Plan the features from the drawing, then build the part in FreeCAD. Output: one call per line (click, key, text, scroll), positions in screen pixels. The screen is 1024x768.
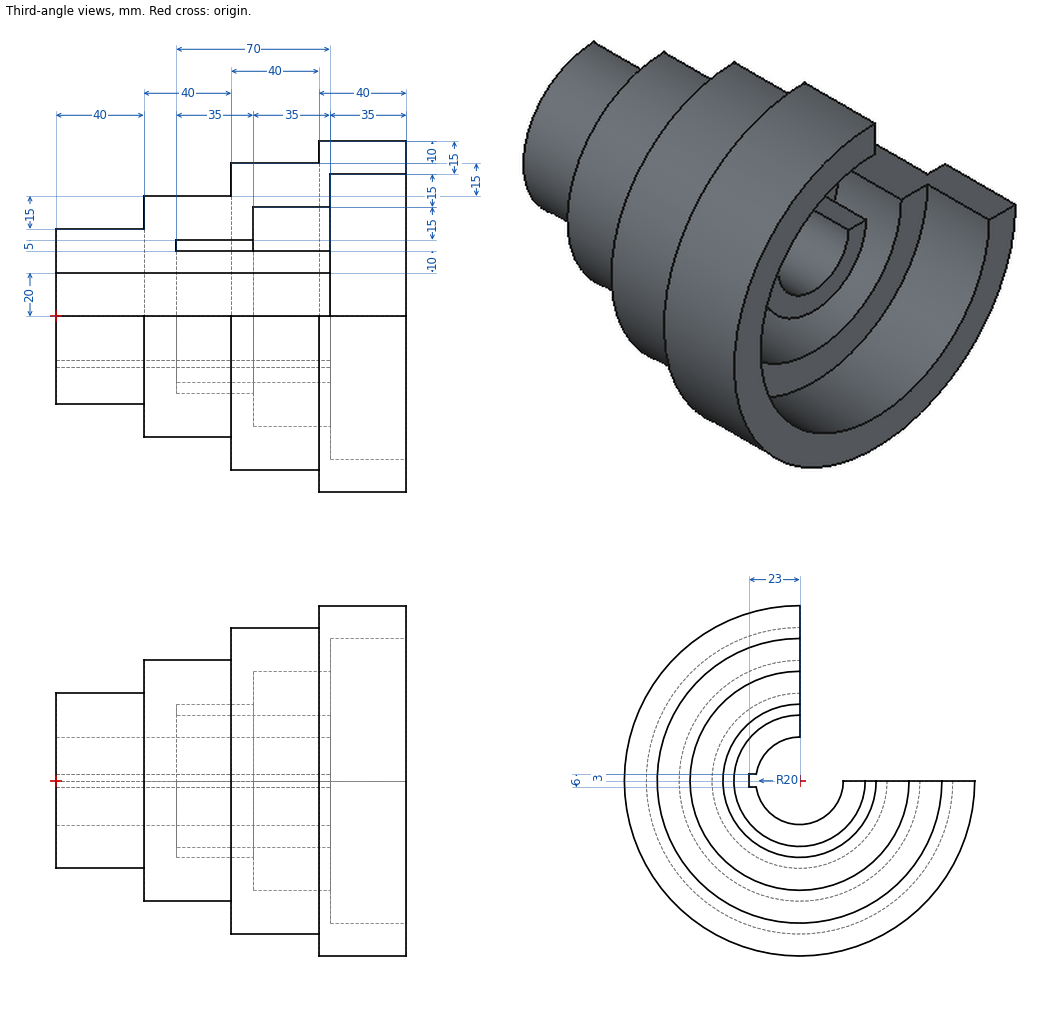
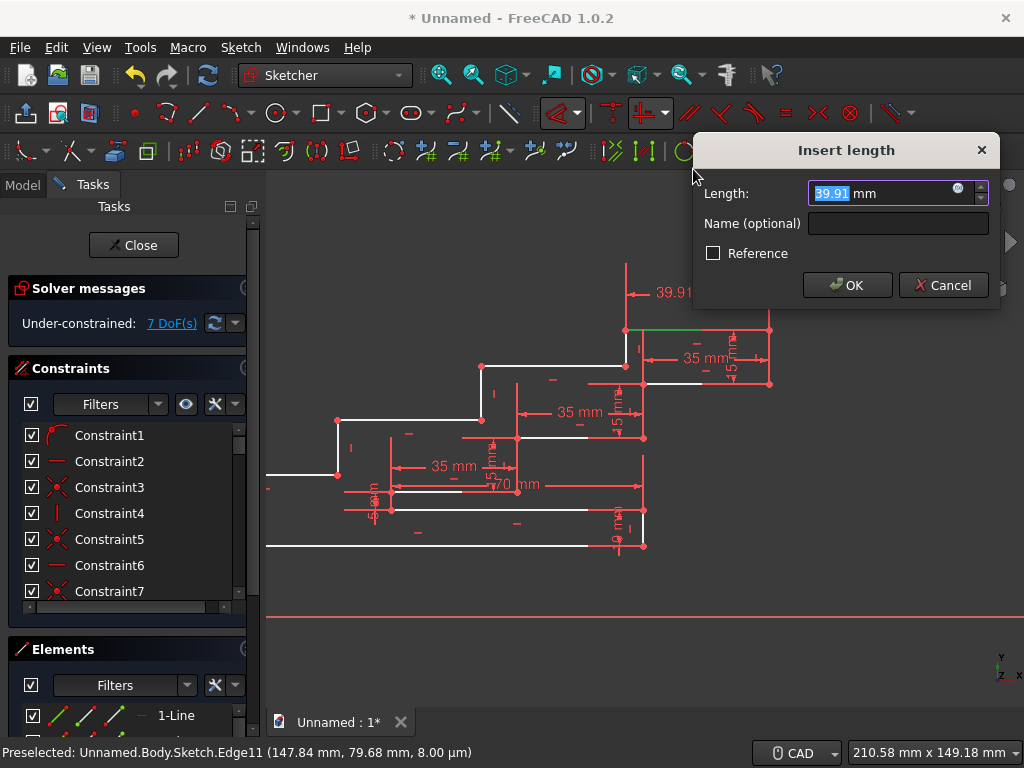
text(40)
key(Return)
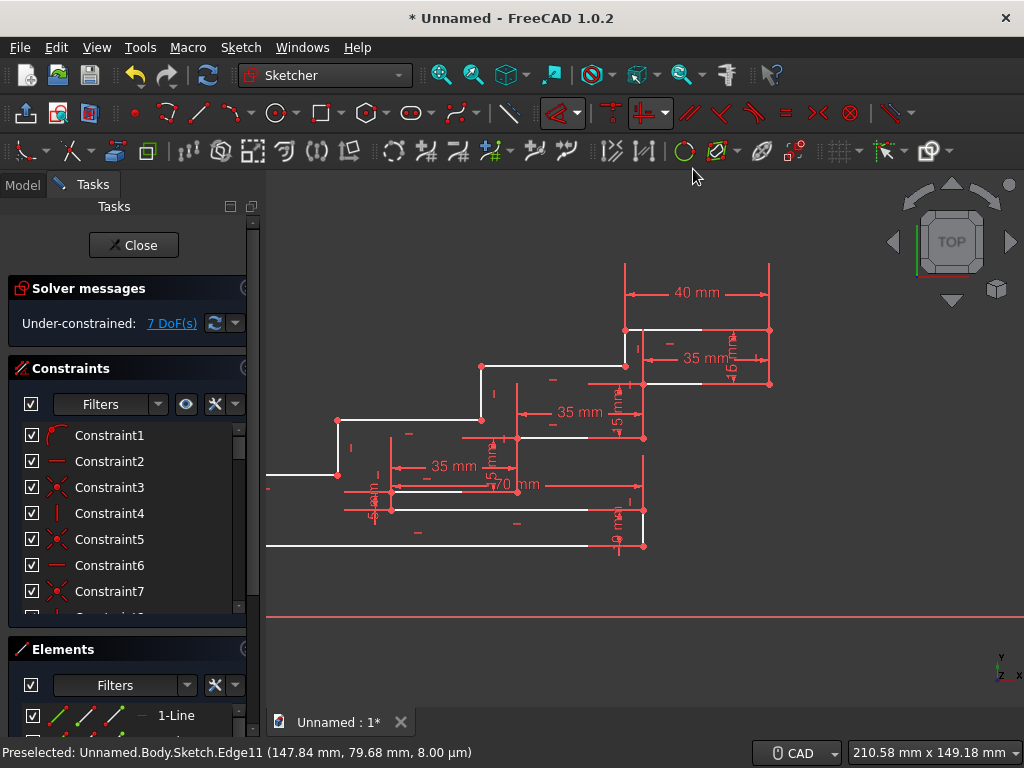
scroll(625, 341, up, 2)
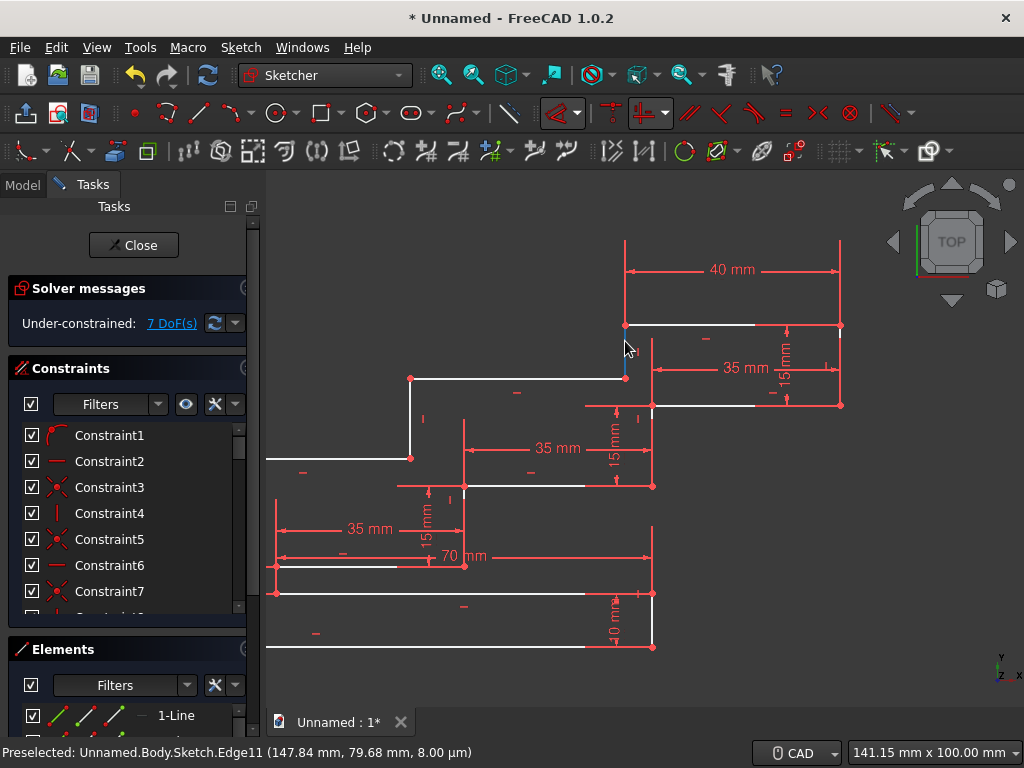
click(625, 341)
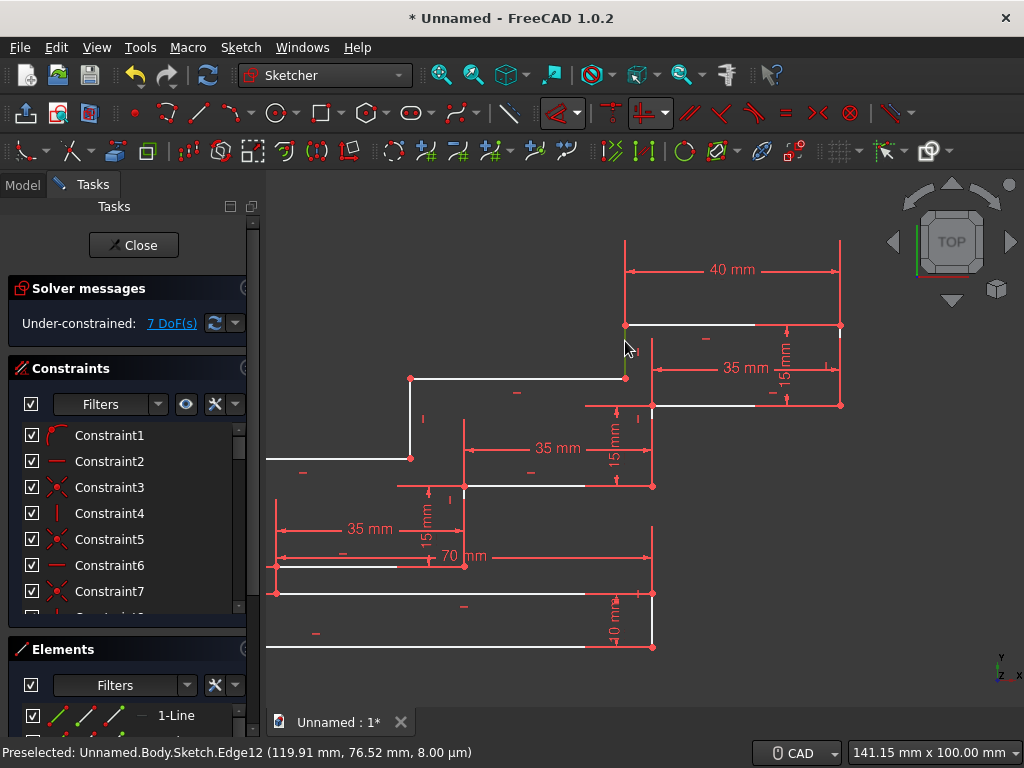
click(580, 114)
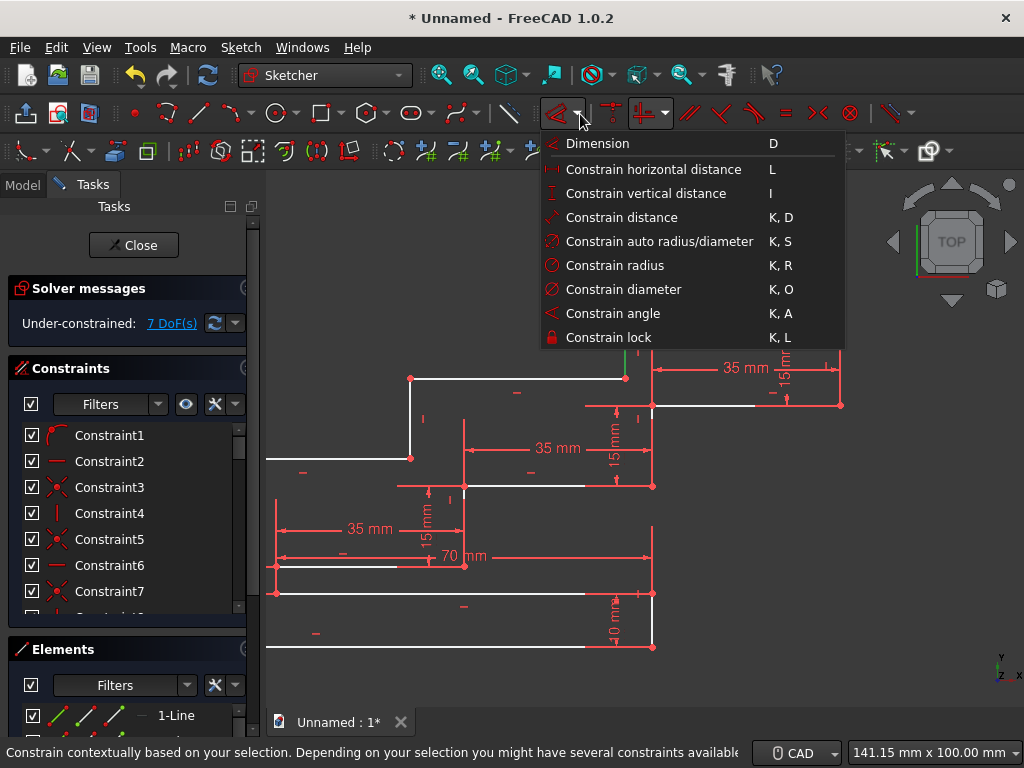
click(693, 193)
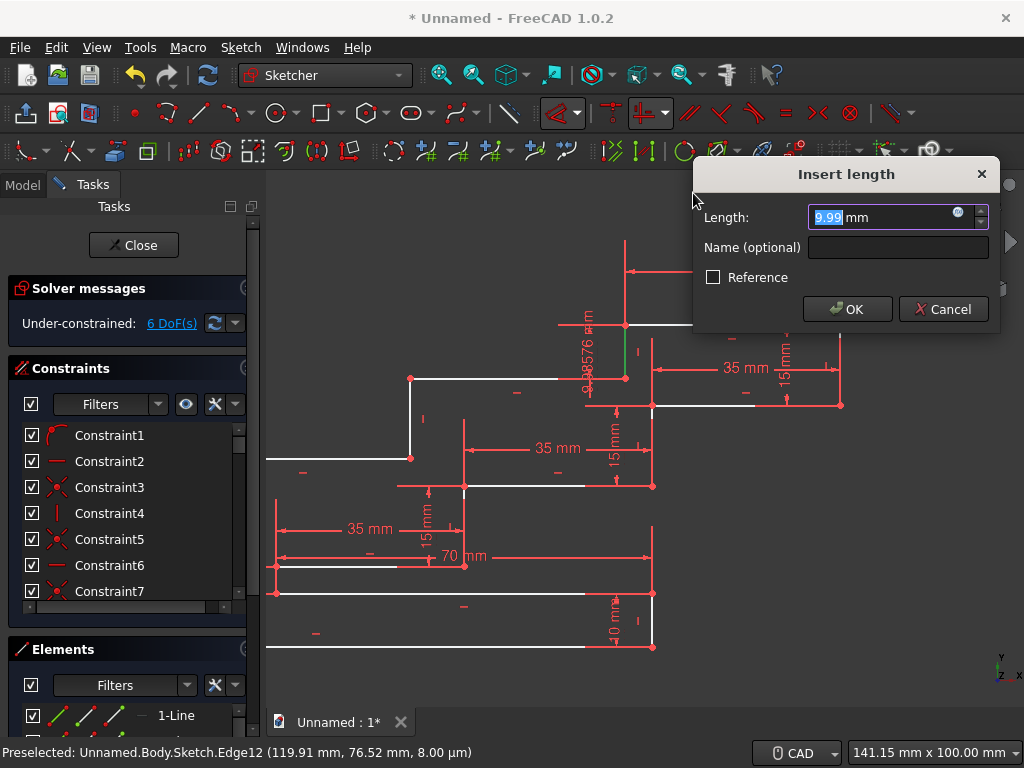
text(10)
key(Return)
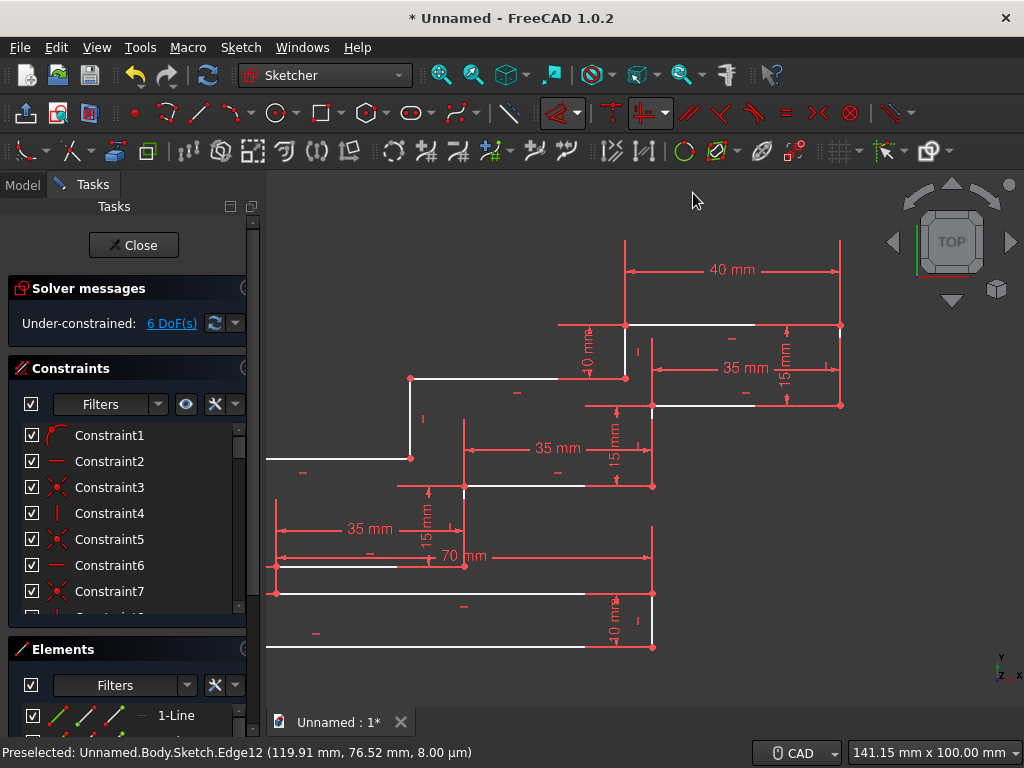
click(561, 379)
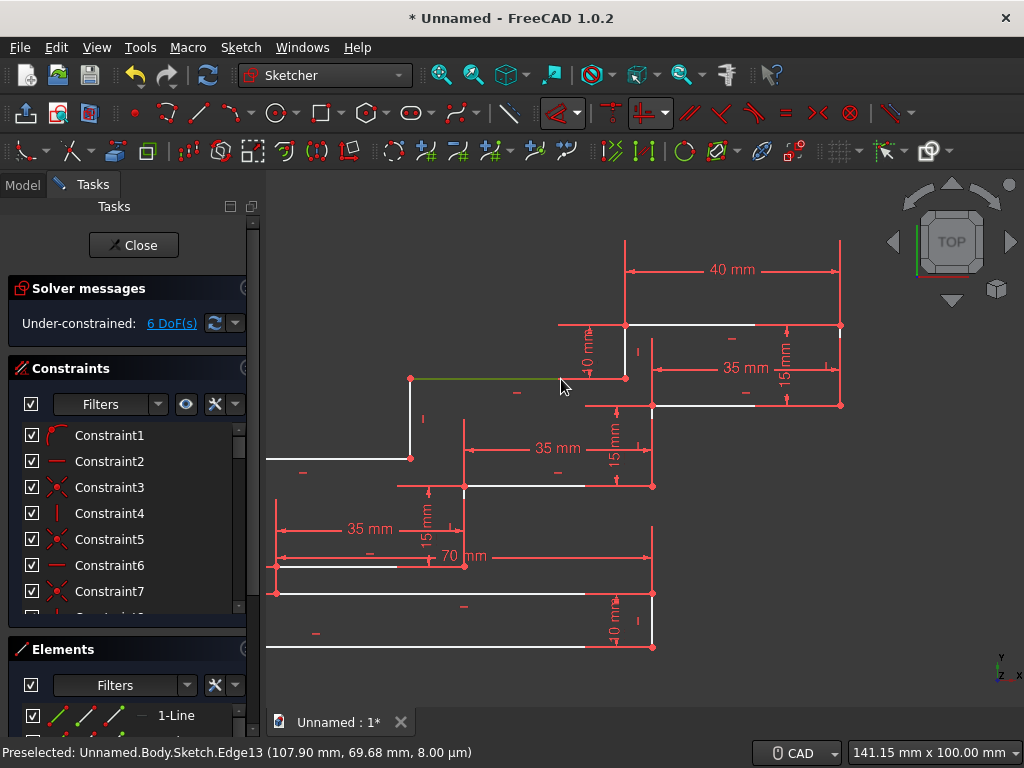
key(l)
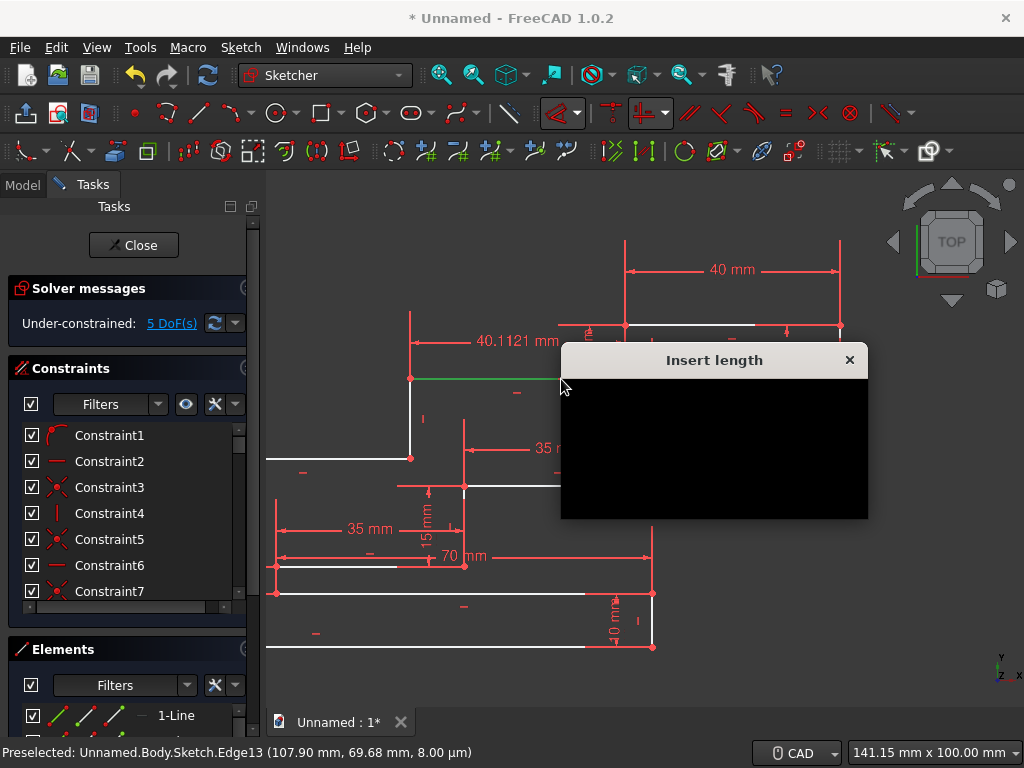
text(40)
key(Return)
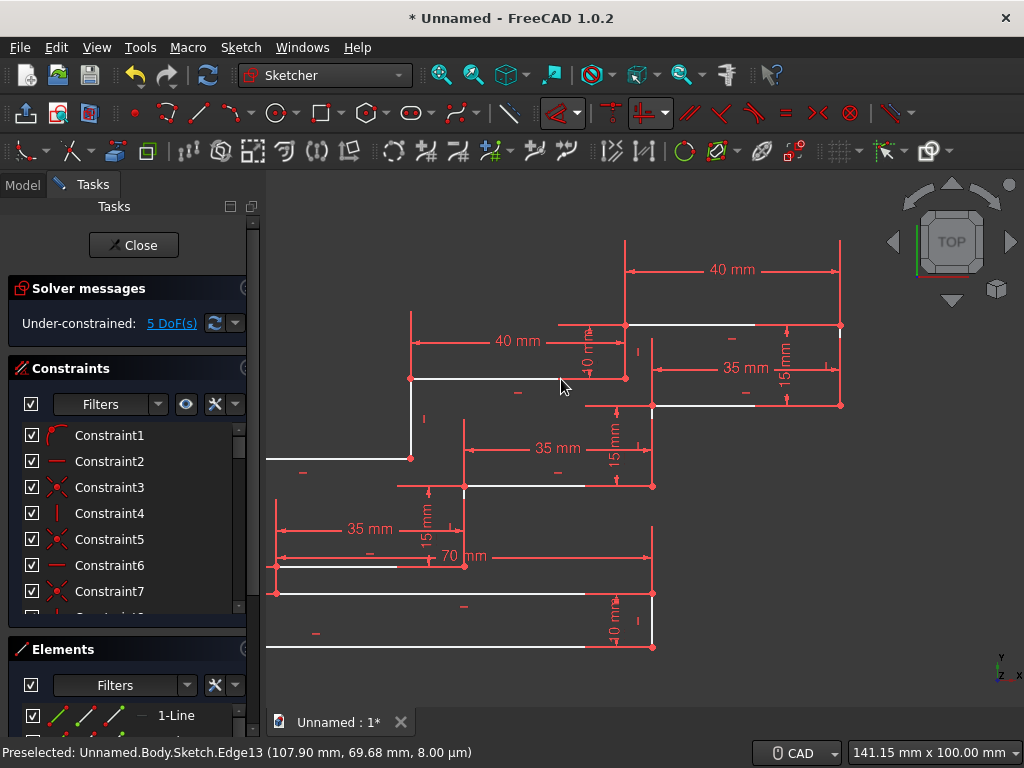
click(411, 403)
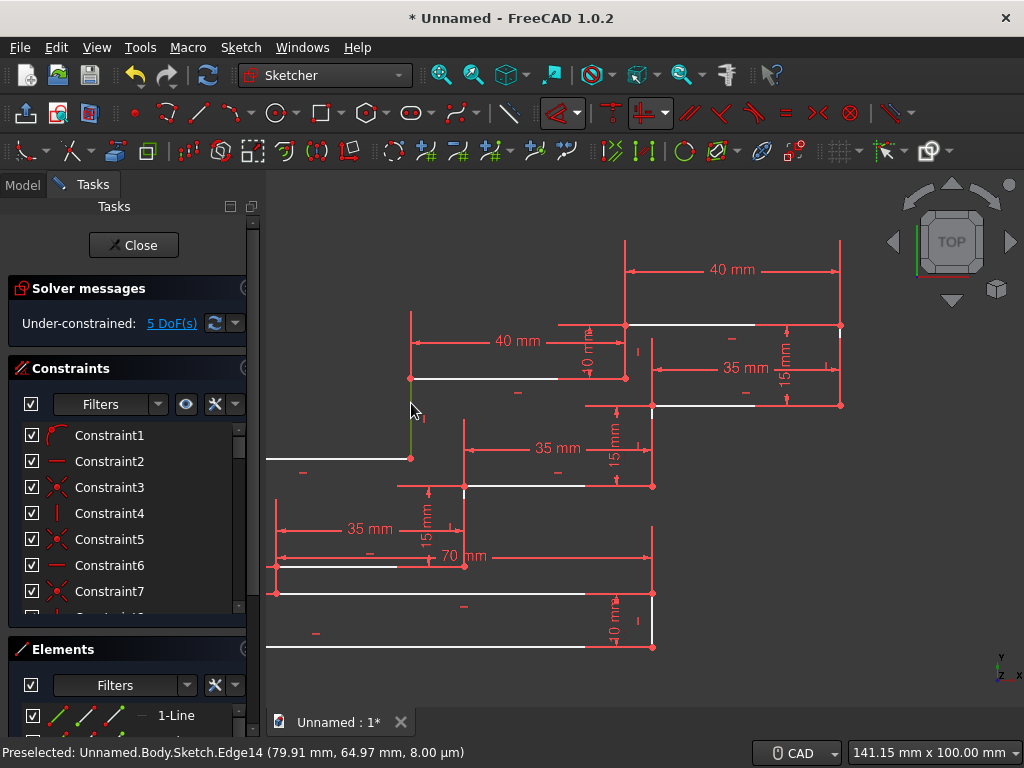
click(580, 114)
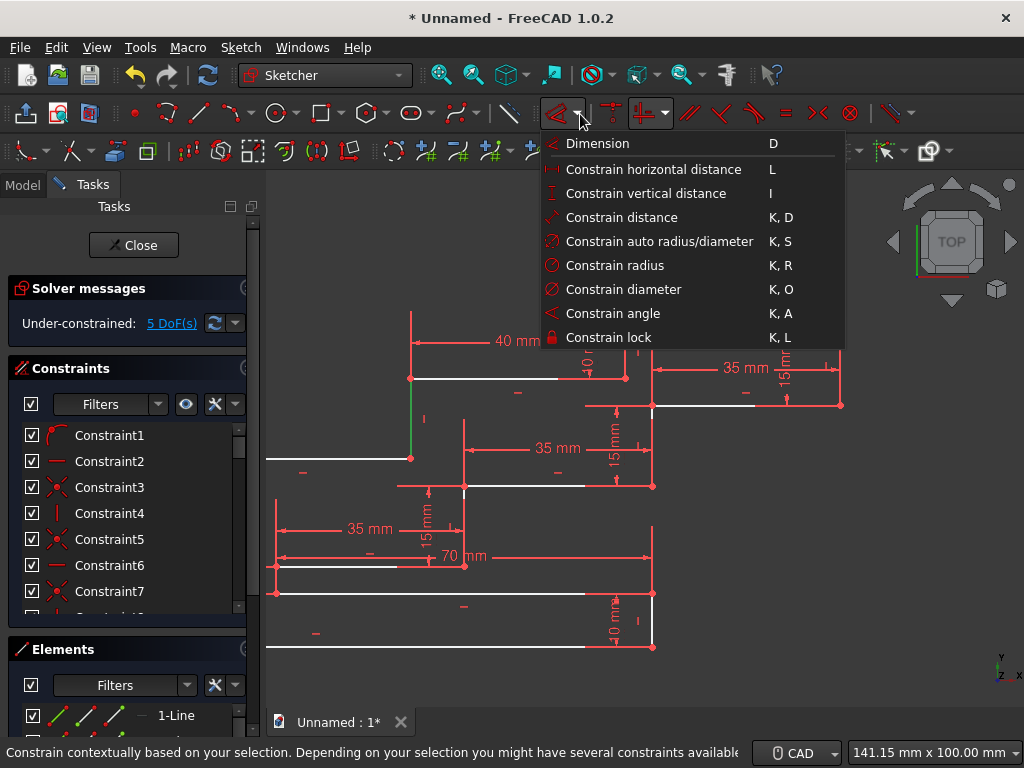
click(693, 193)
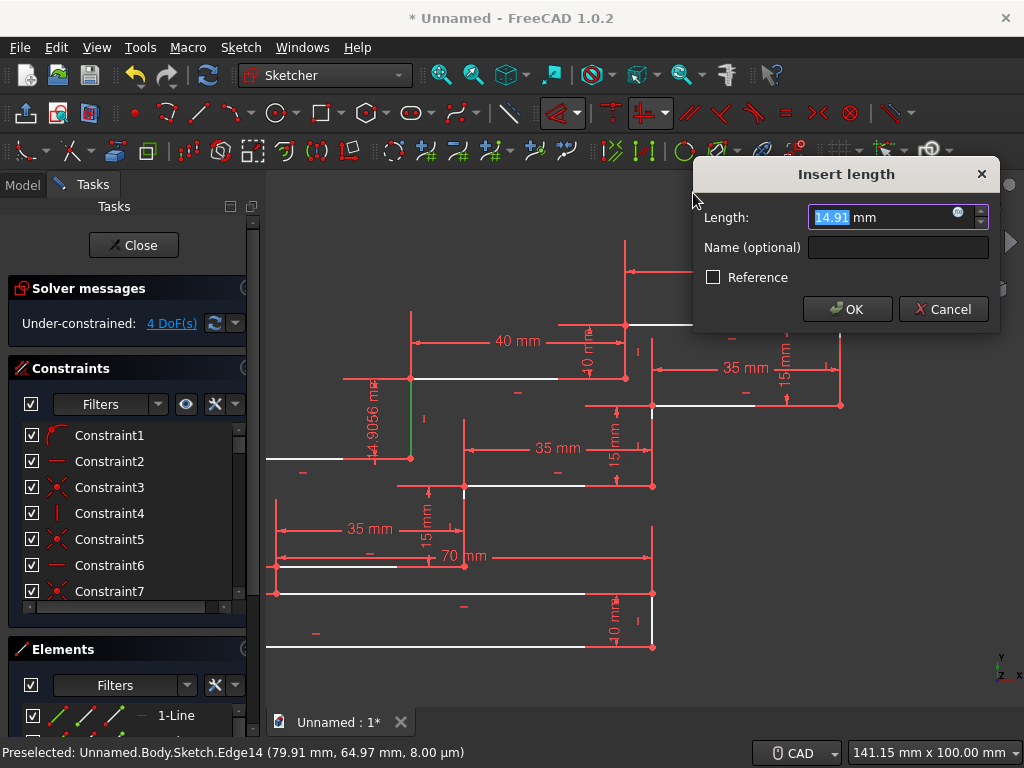
text(15)
key(Return)